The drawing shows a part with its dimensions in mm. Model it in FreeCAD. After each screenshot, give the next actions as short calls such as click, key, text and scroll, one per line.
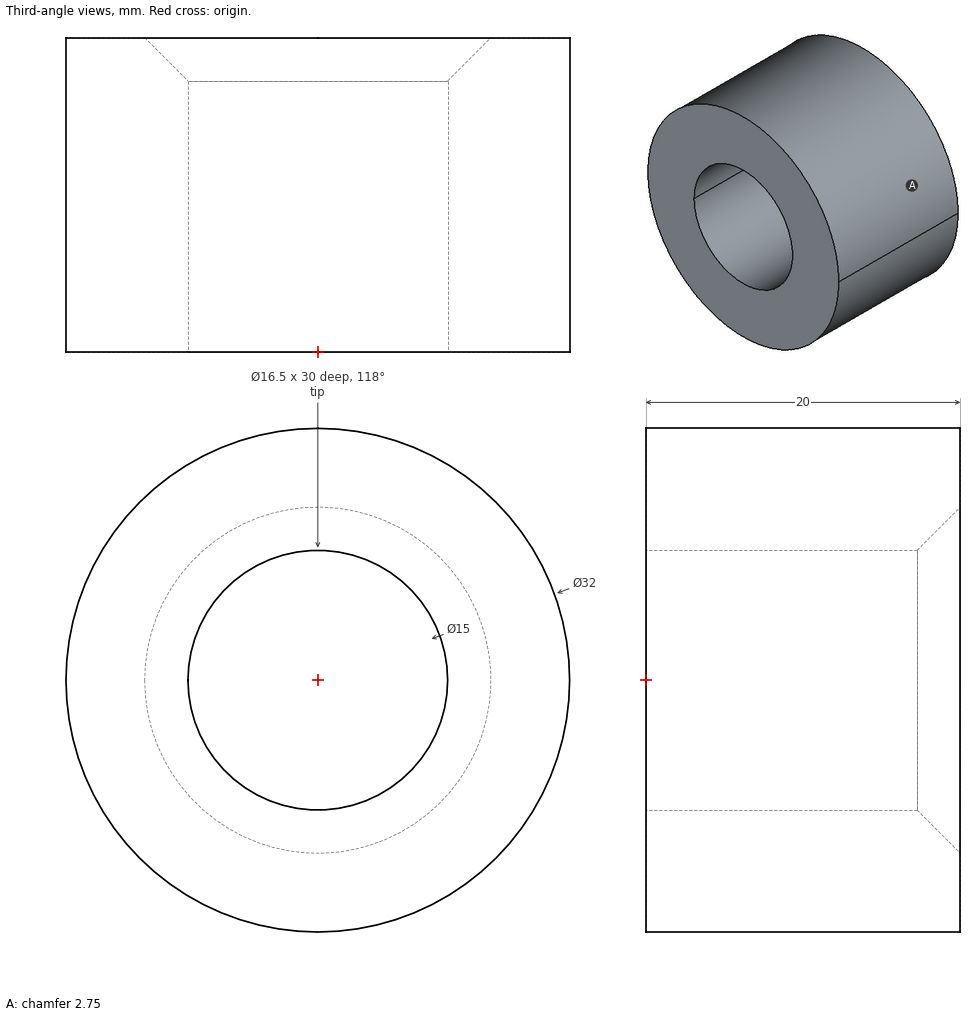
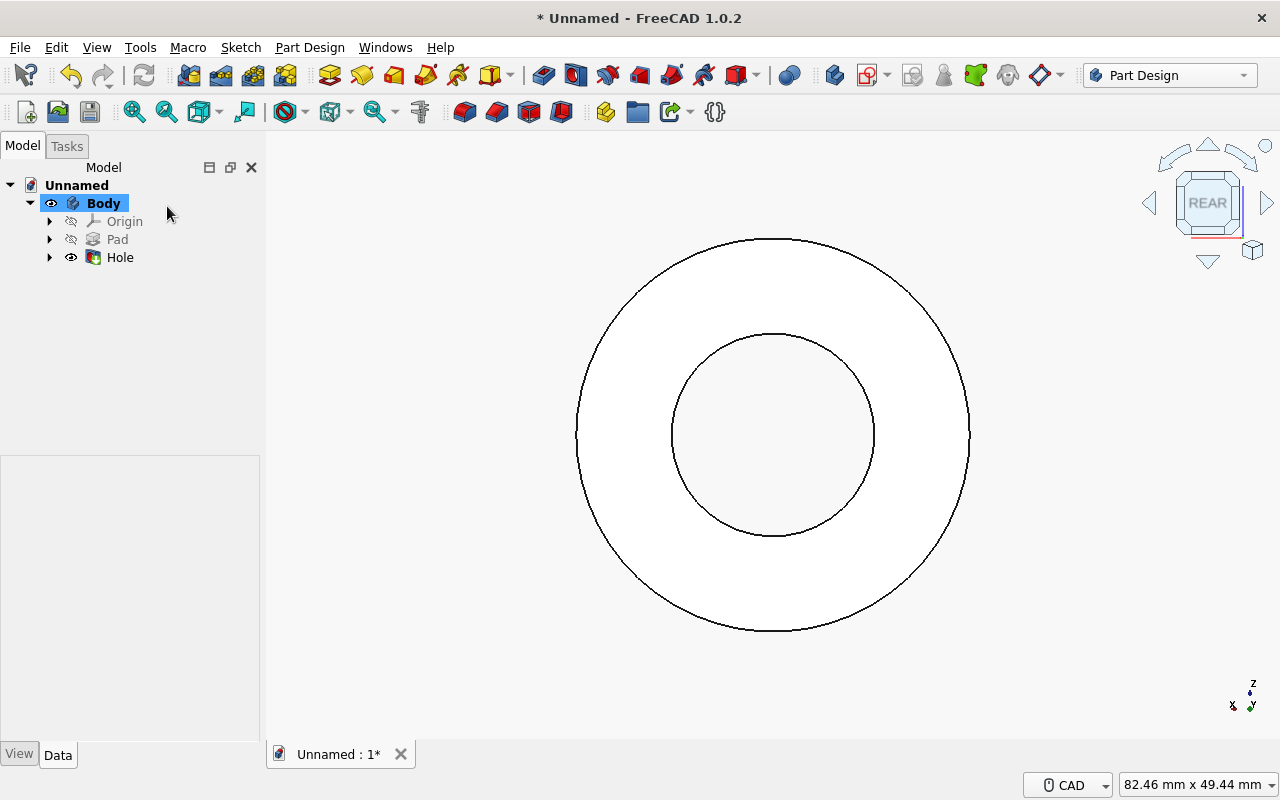
click(672, 434)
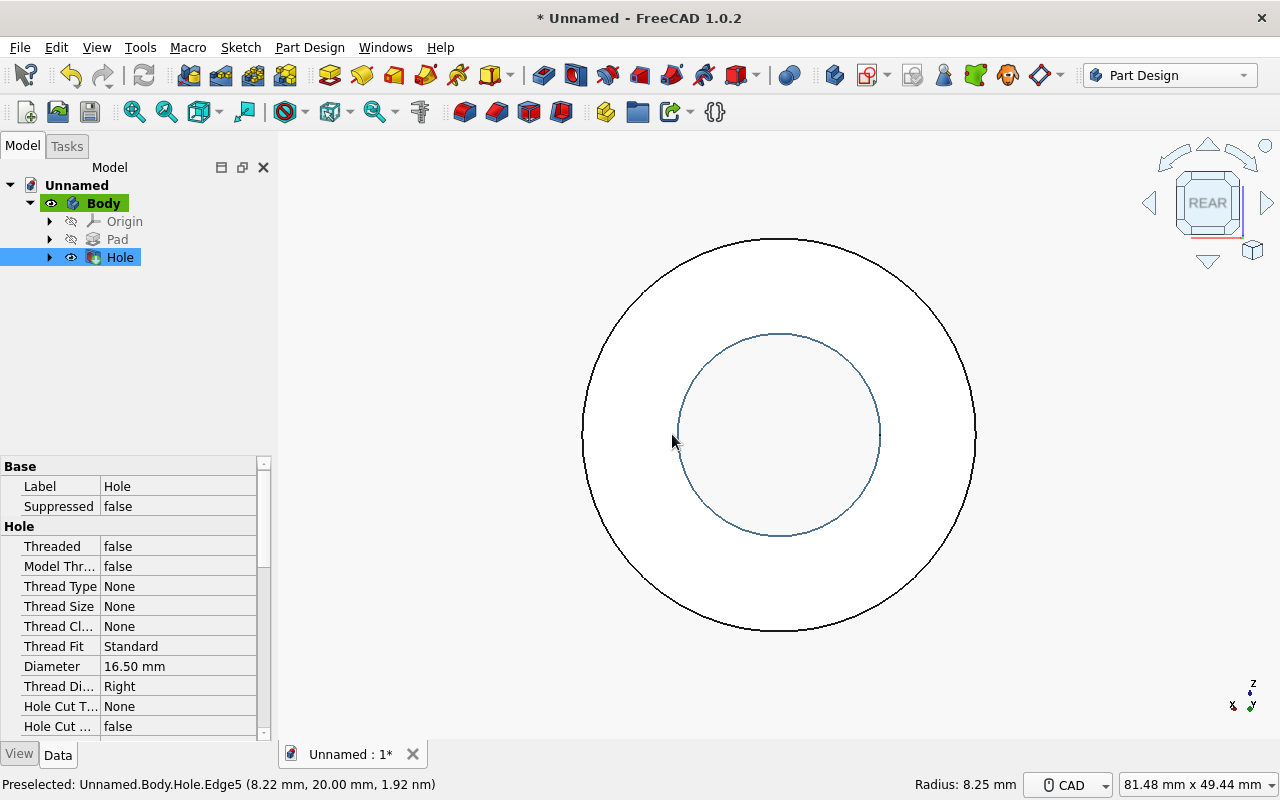
click(498, 112)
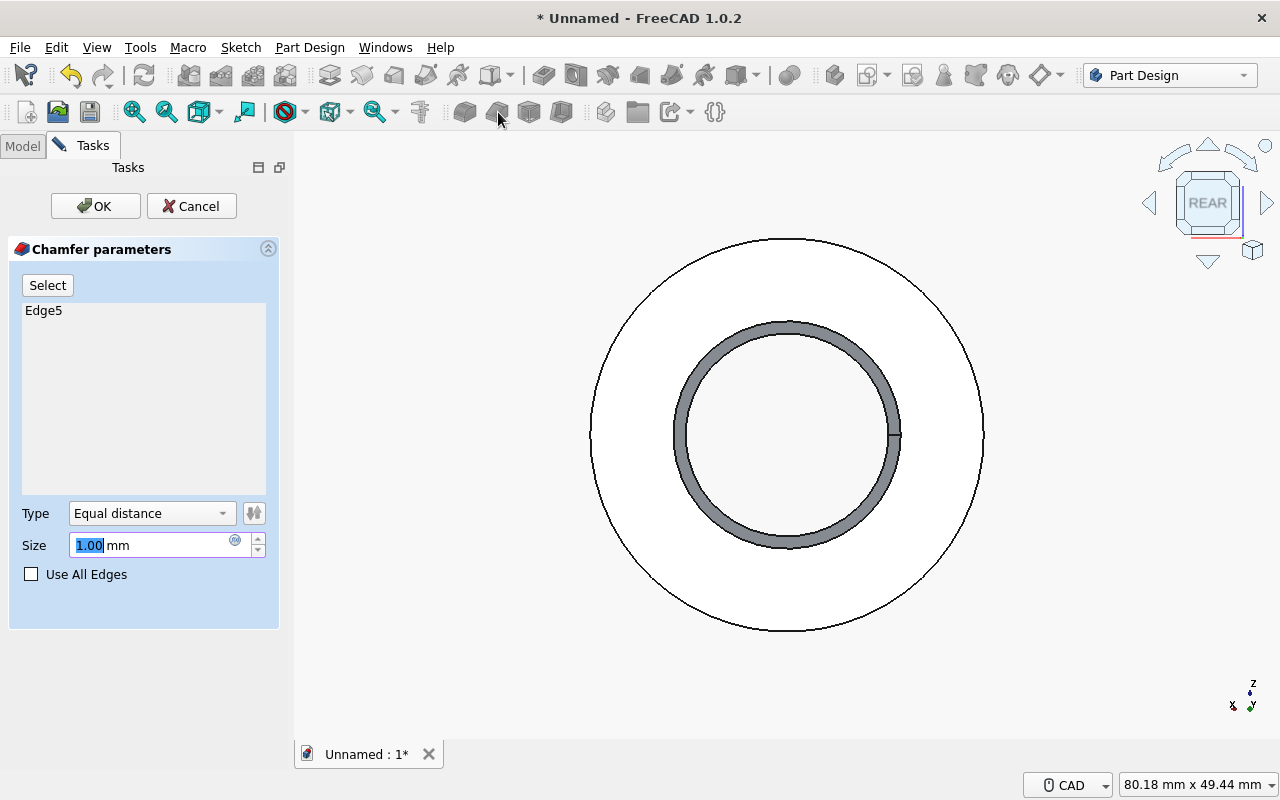
text(2.75)
key(Tab)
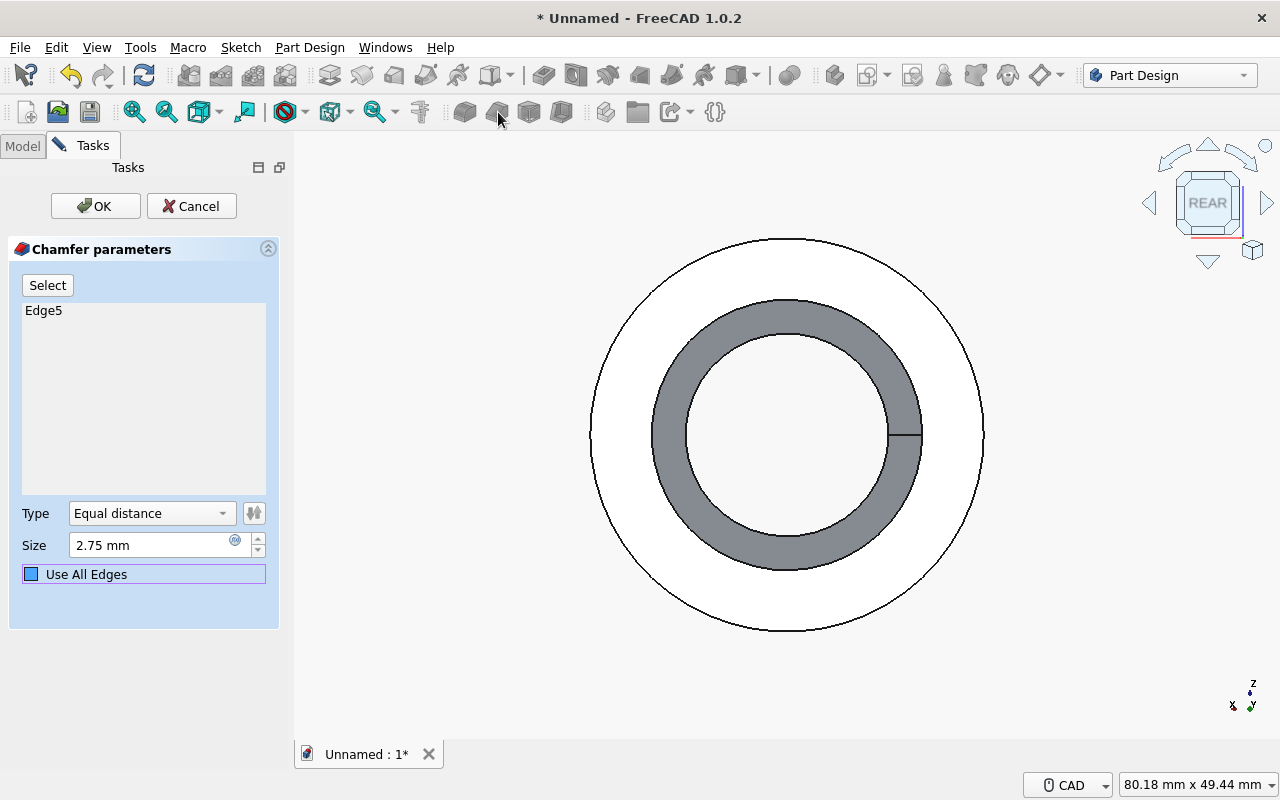
click(96, 206)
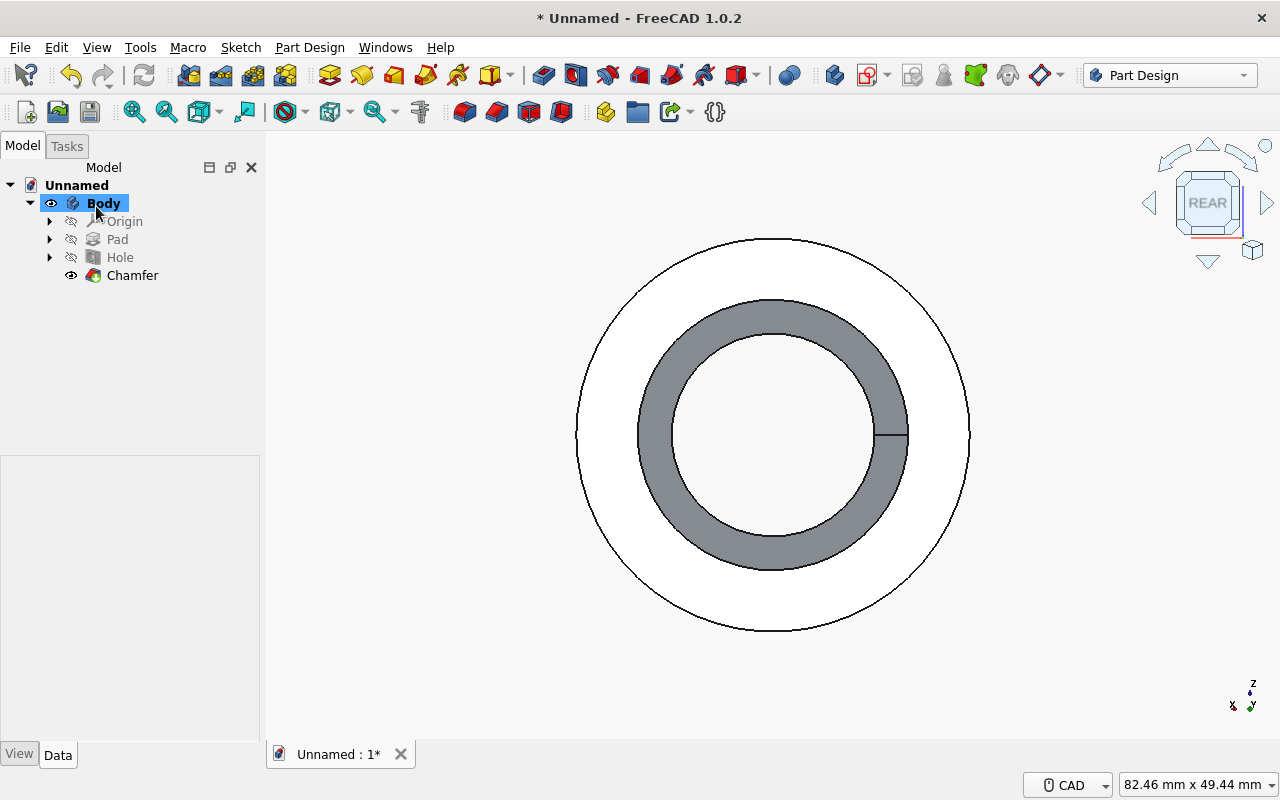
key(0)